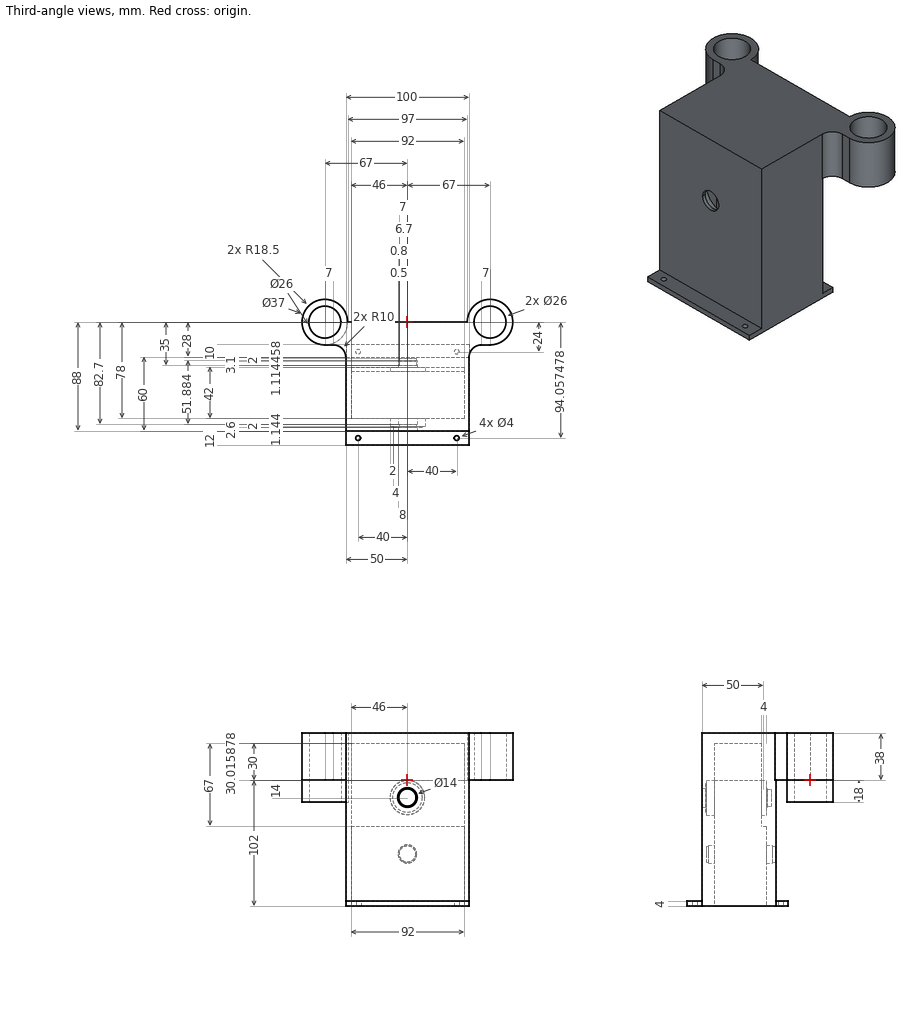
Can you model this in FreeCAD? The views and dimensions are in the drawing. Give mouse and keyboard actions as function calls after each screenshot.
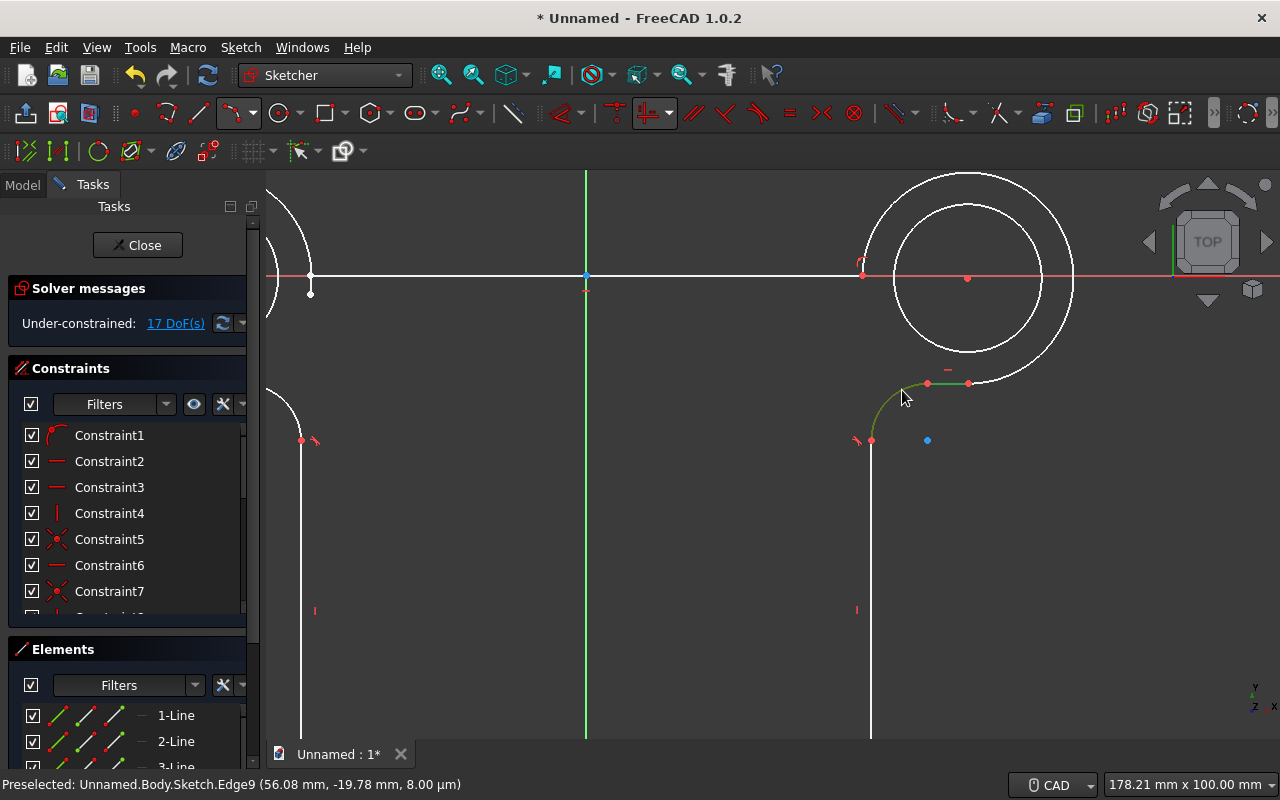
key(t)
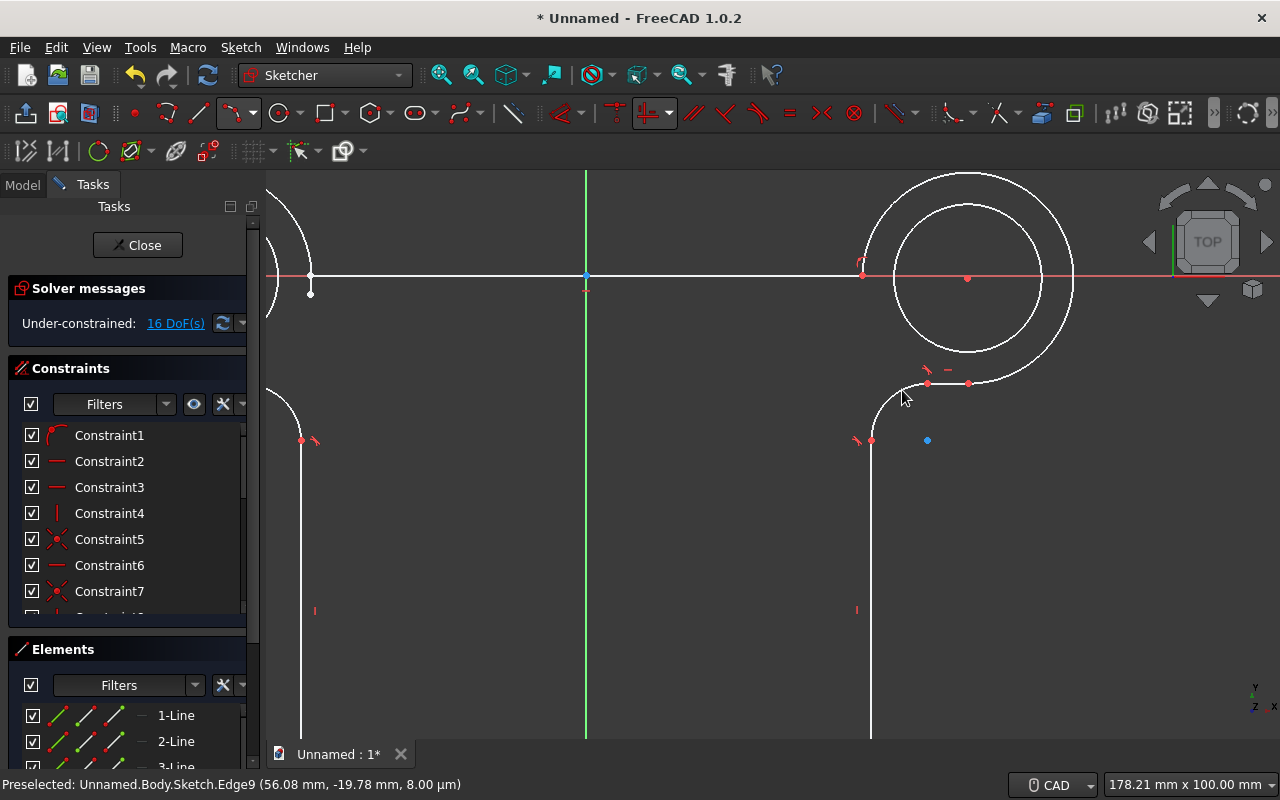
click(940, 384)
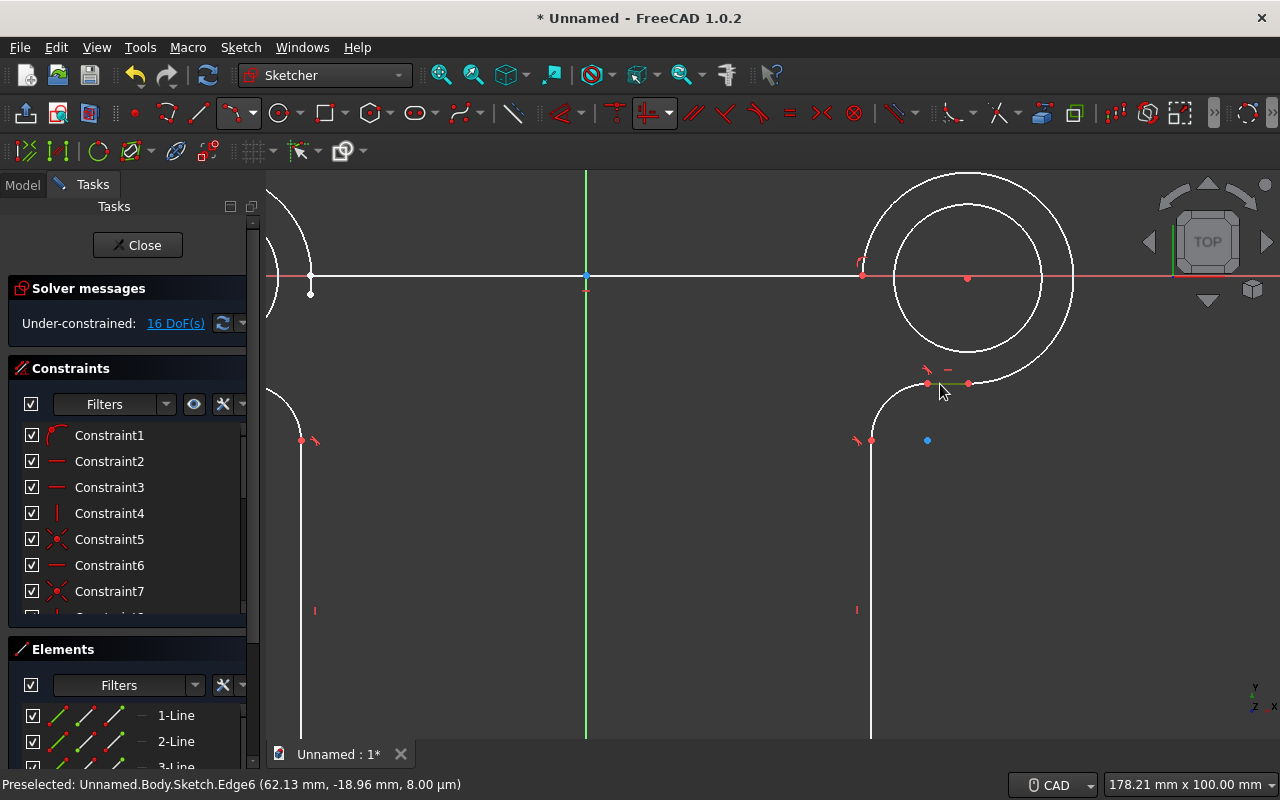
click(1072, 295)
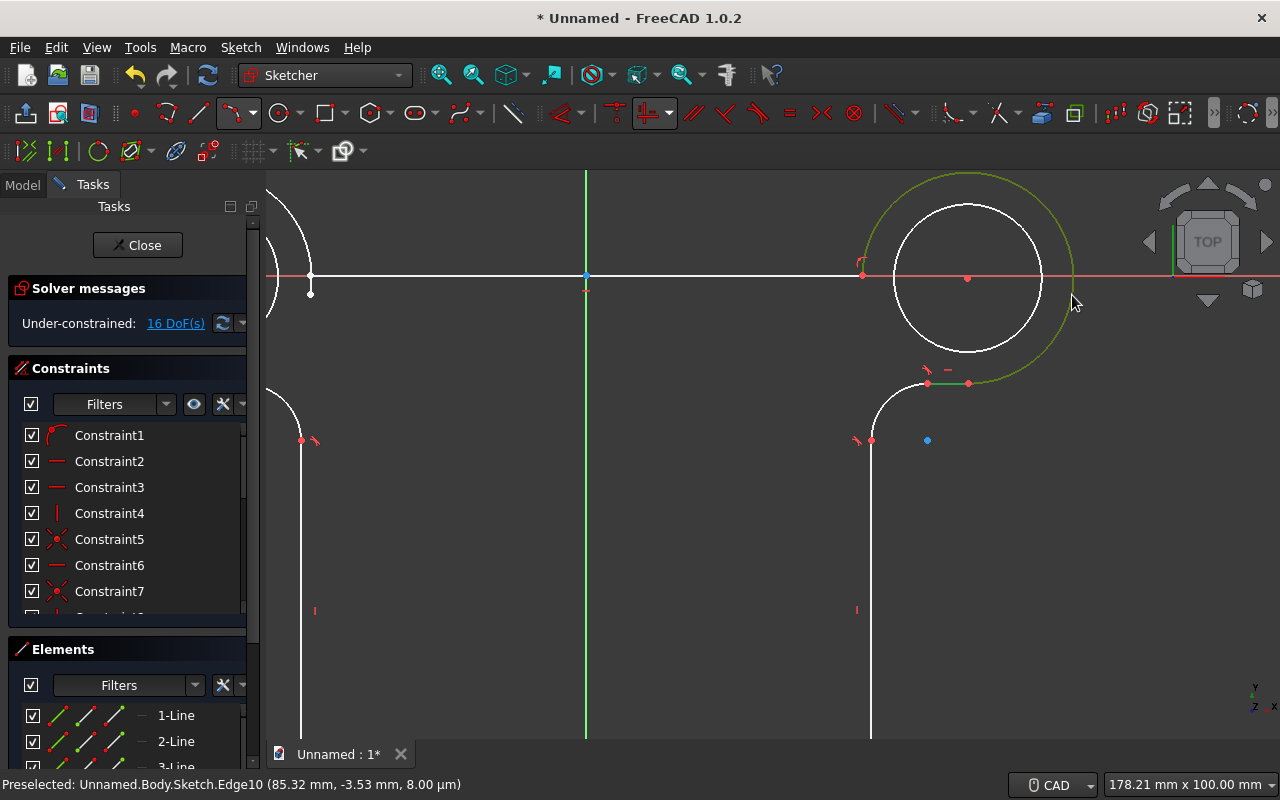
click(758, 114)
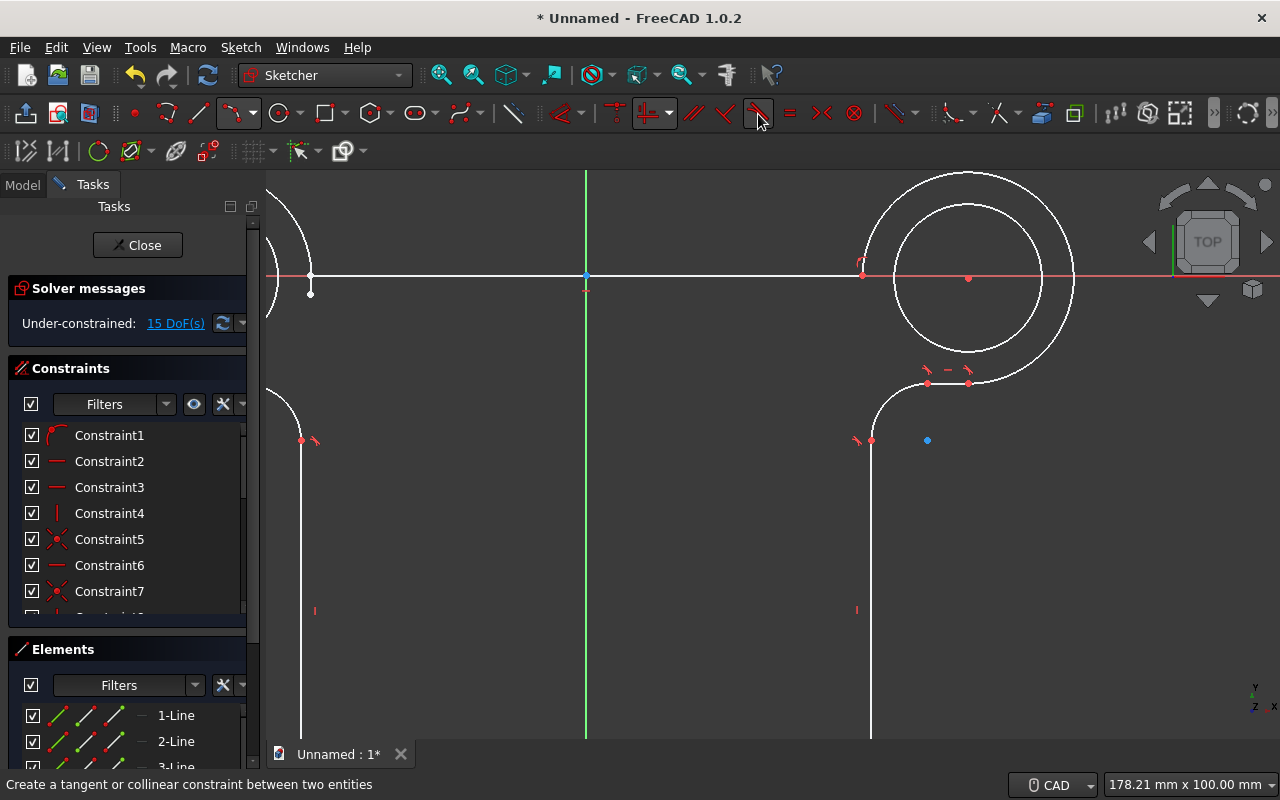
click(295, 415)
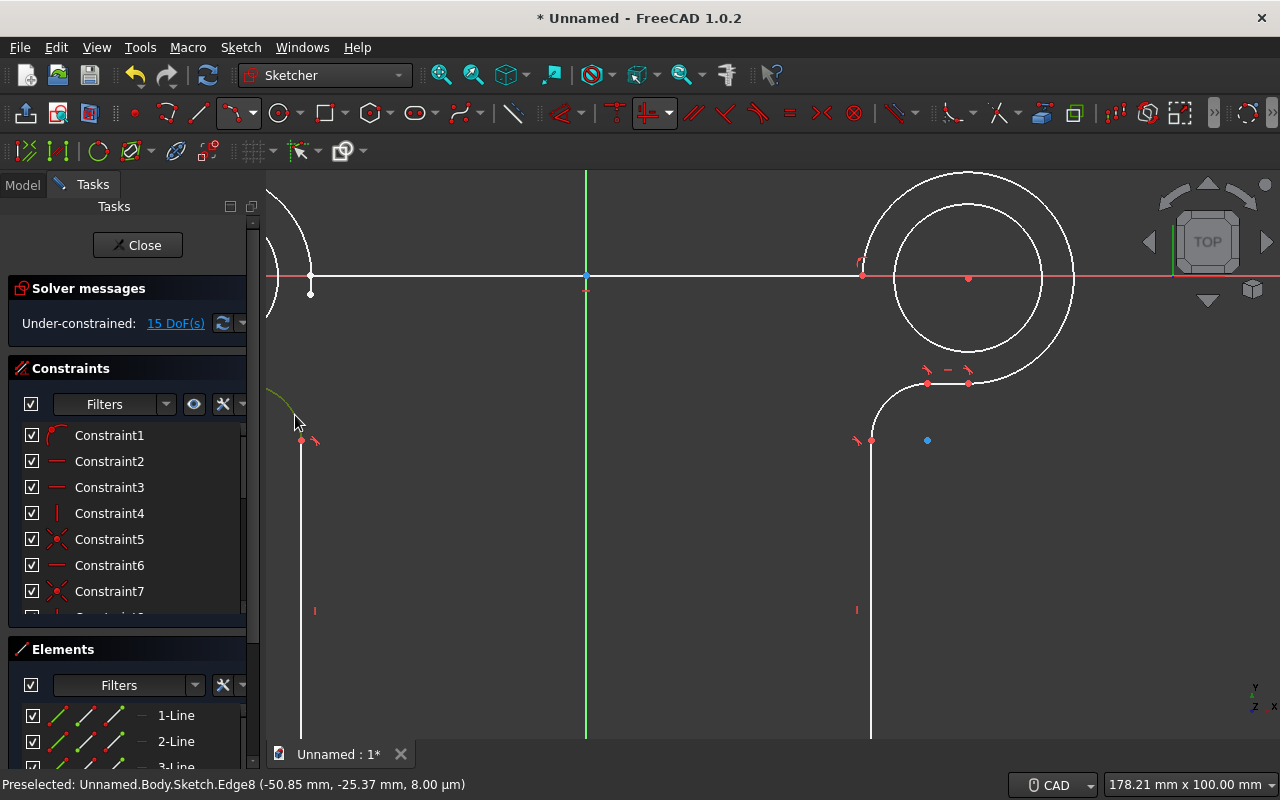
click(902, 390)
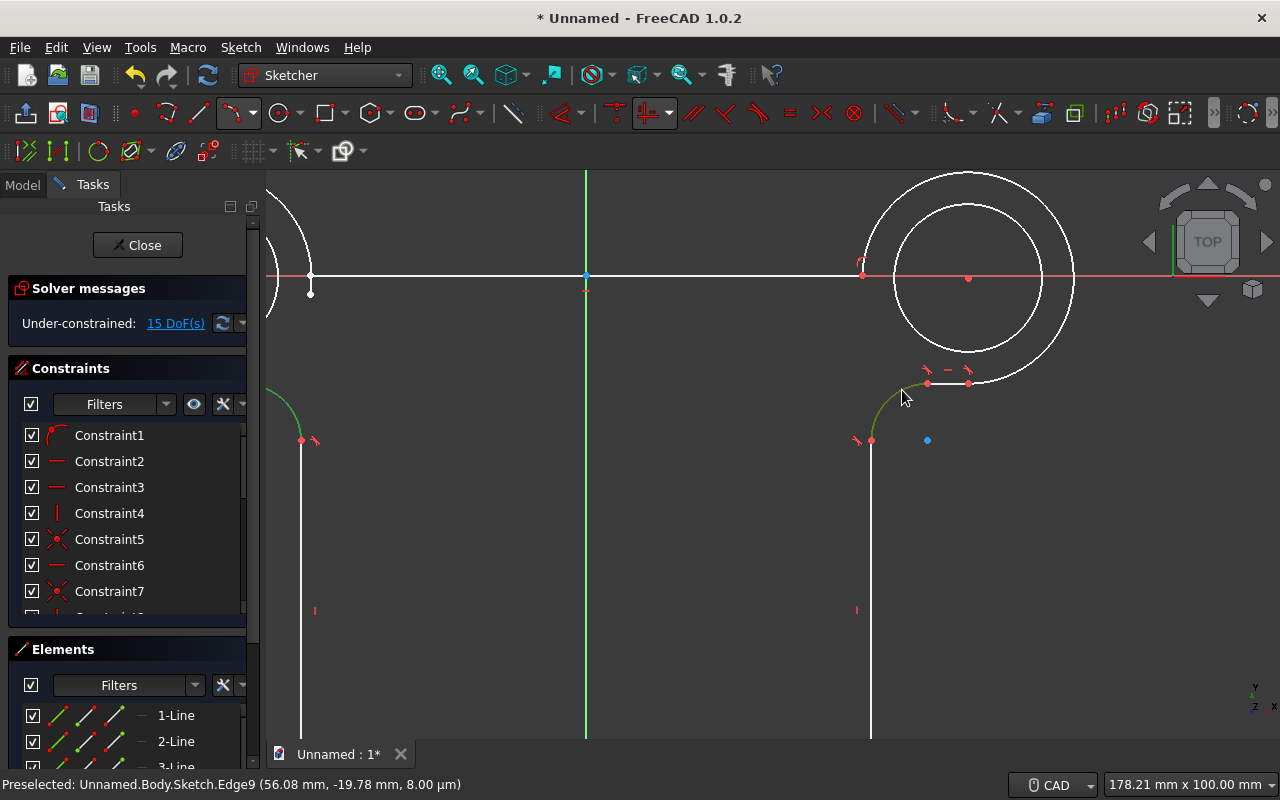
key(e)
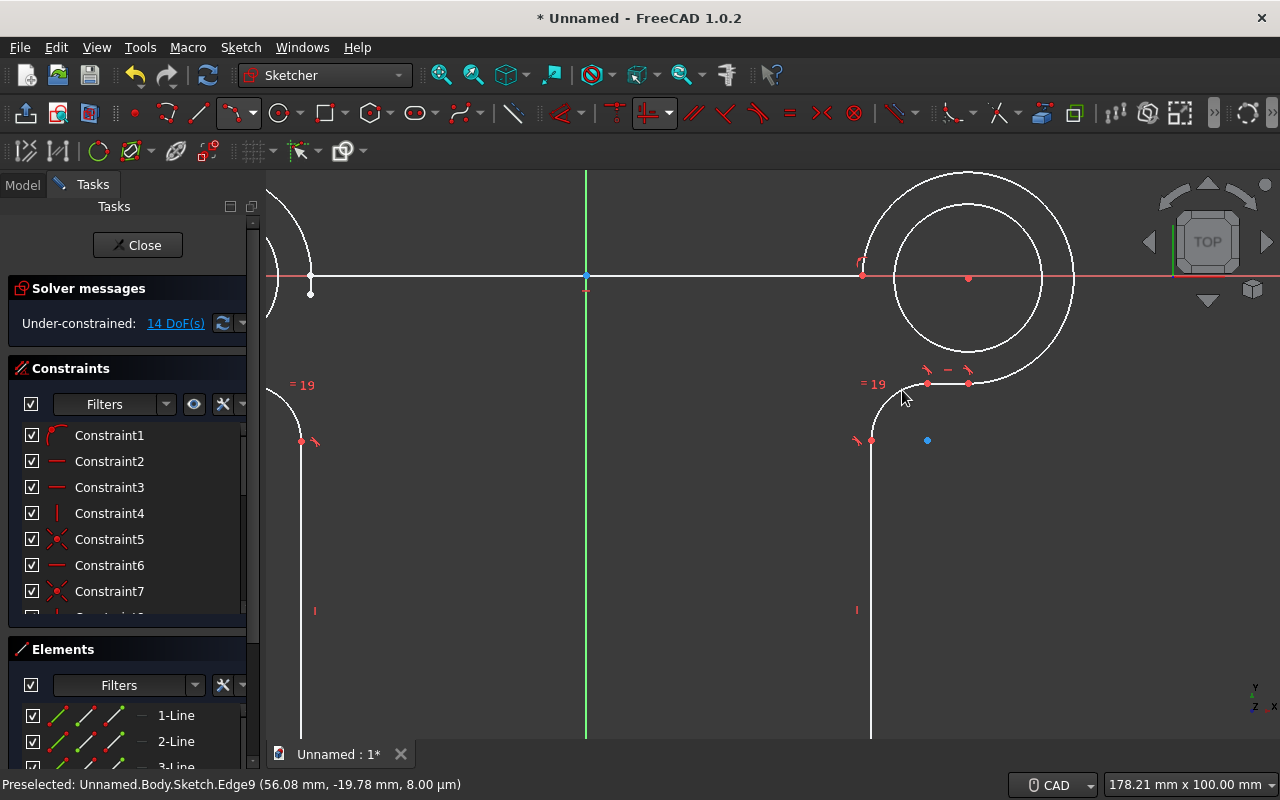
scroll(944, 384, down, 2)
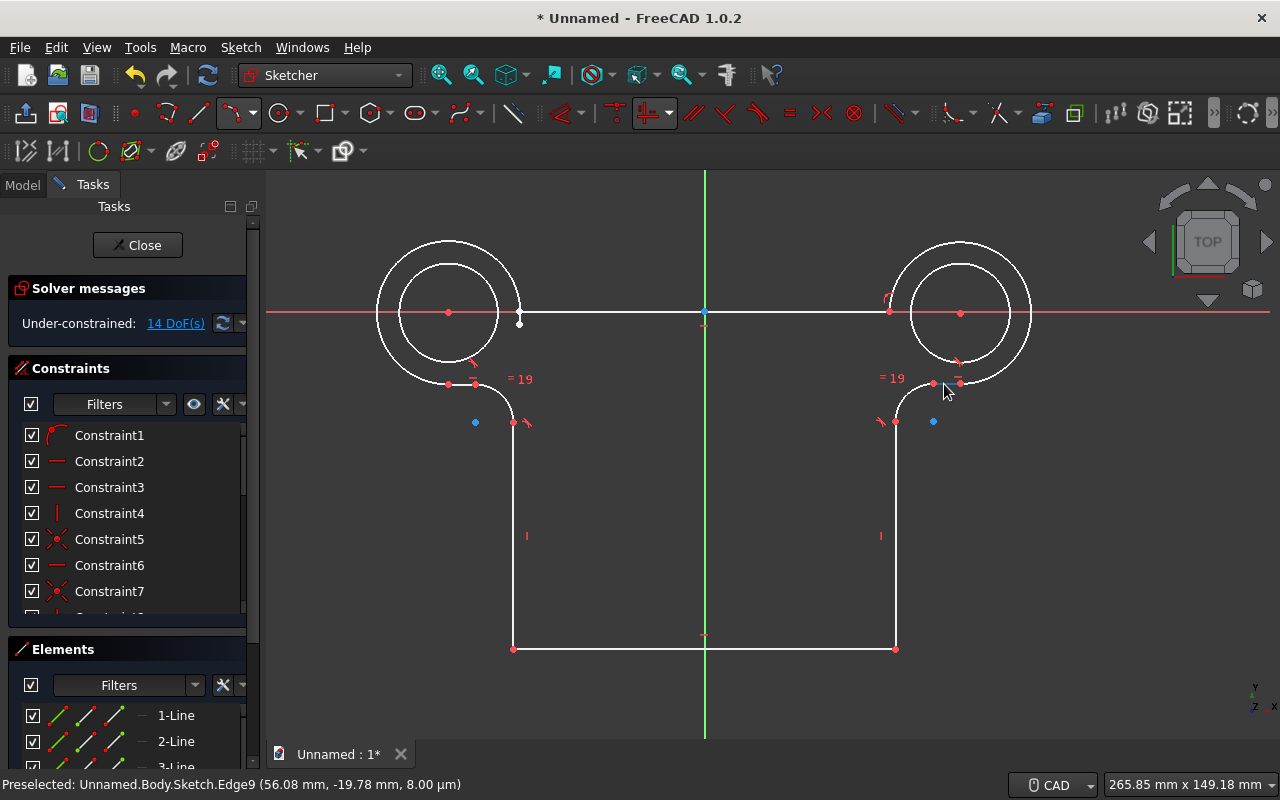
click(468, 244)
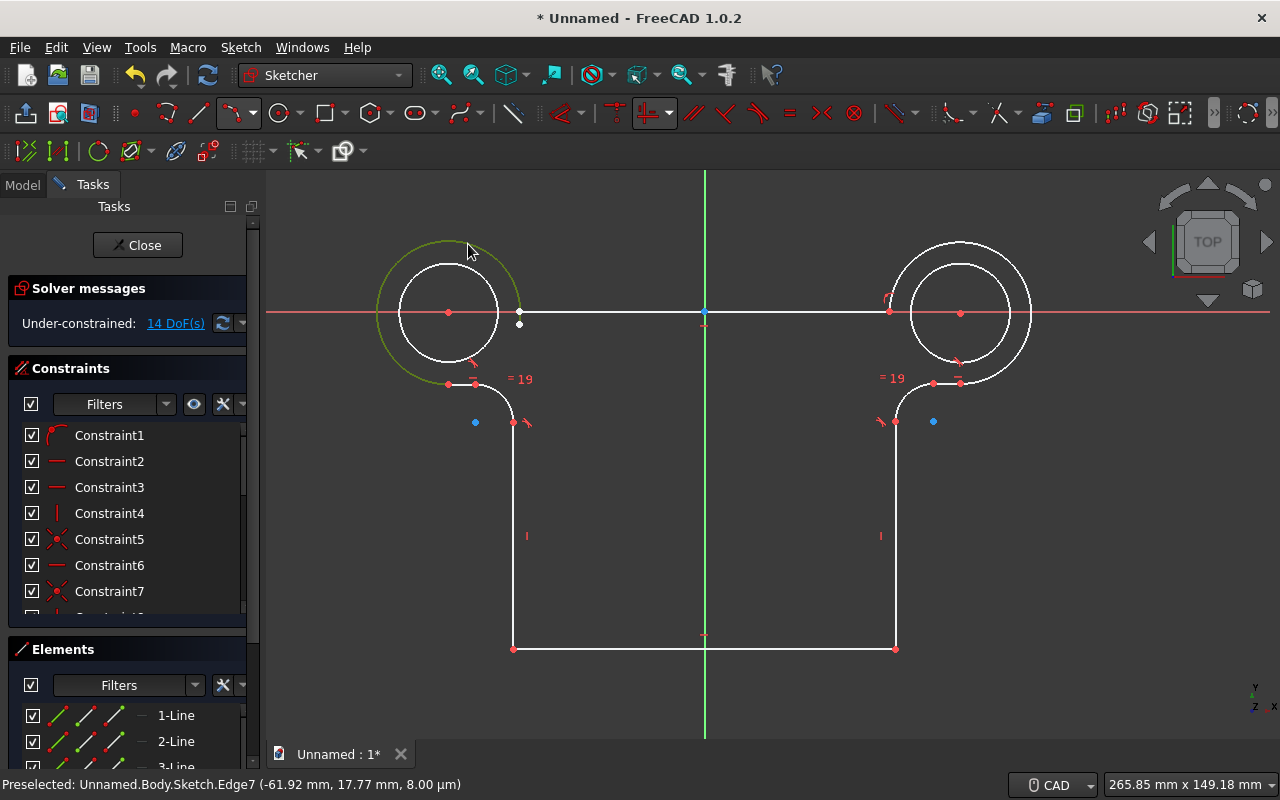
click(1030, 325)